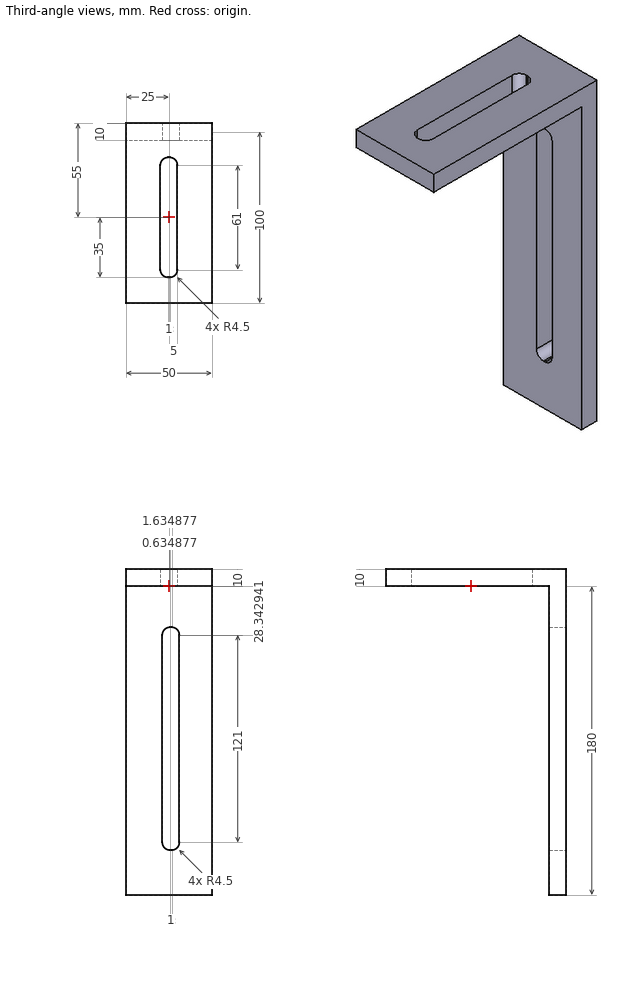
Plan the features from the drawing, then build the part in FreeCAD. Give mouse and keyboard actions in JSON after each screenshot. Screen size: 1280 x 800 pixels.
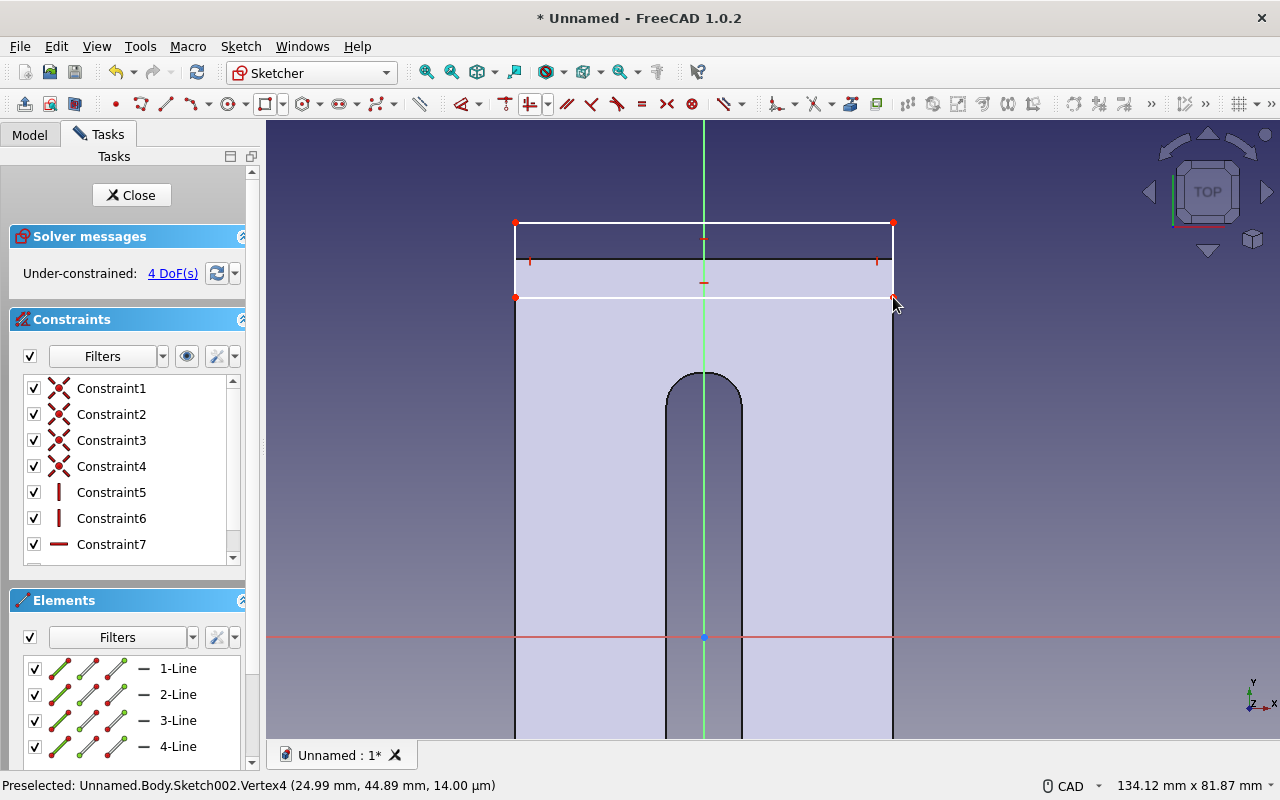
{"action": "left_click", "coordinate": [460, 104]}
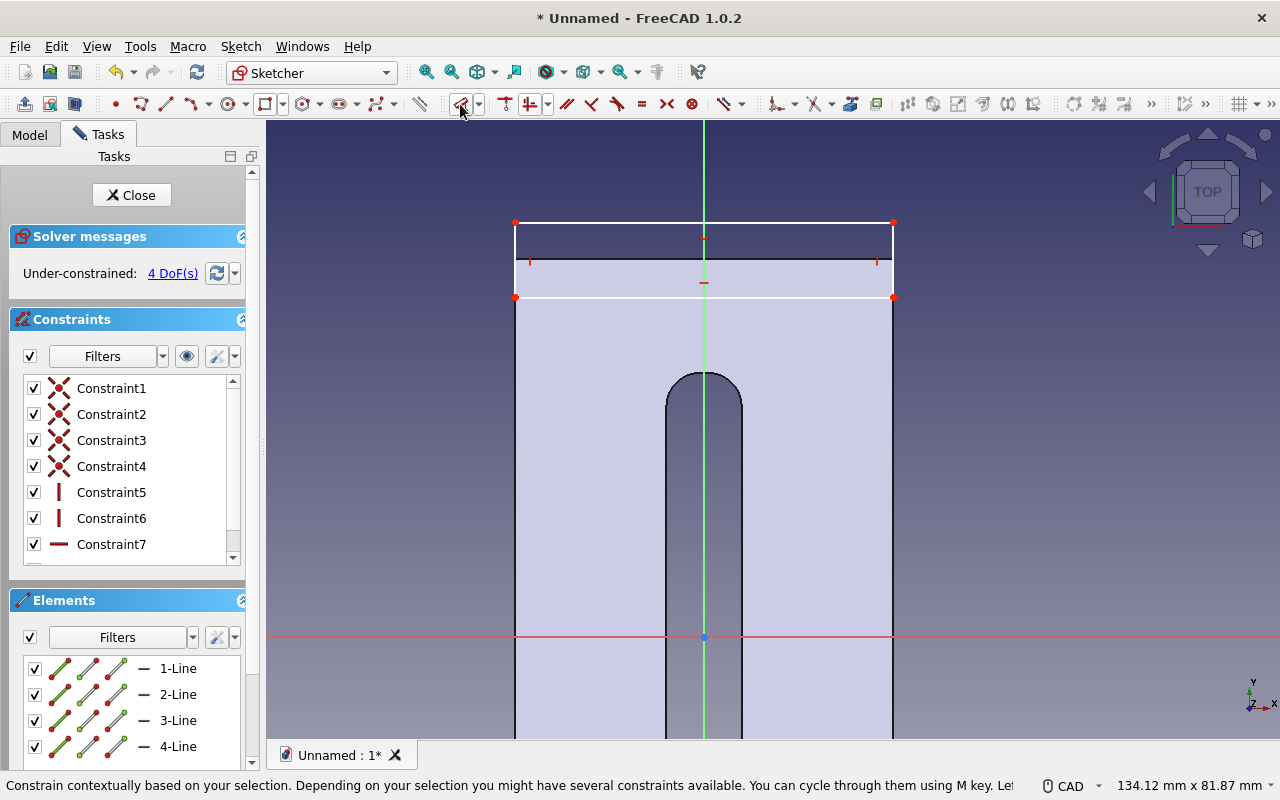
{"action": "left_click", "coordinate": [515, 245]}
{"action": "left_click", "coordinate": [481, 260]}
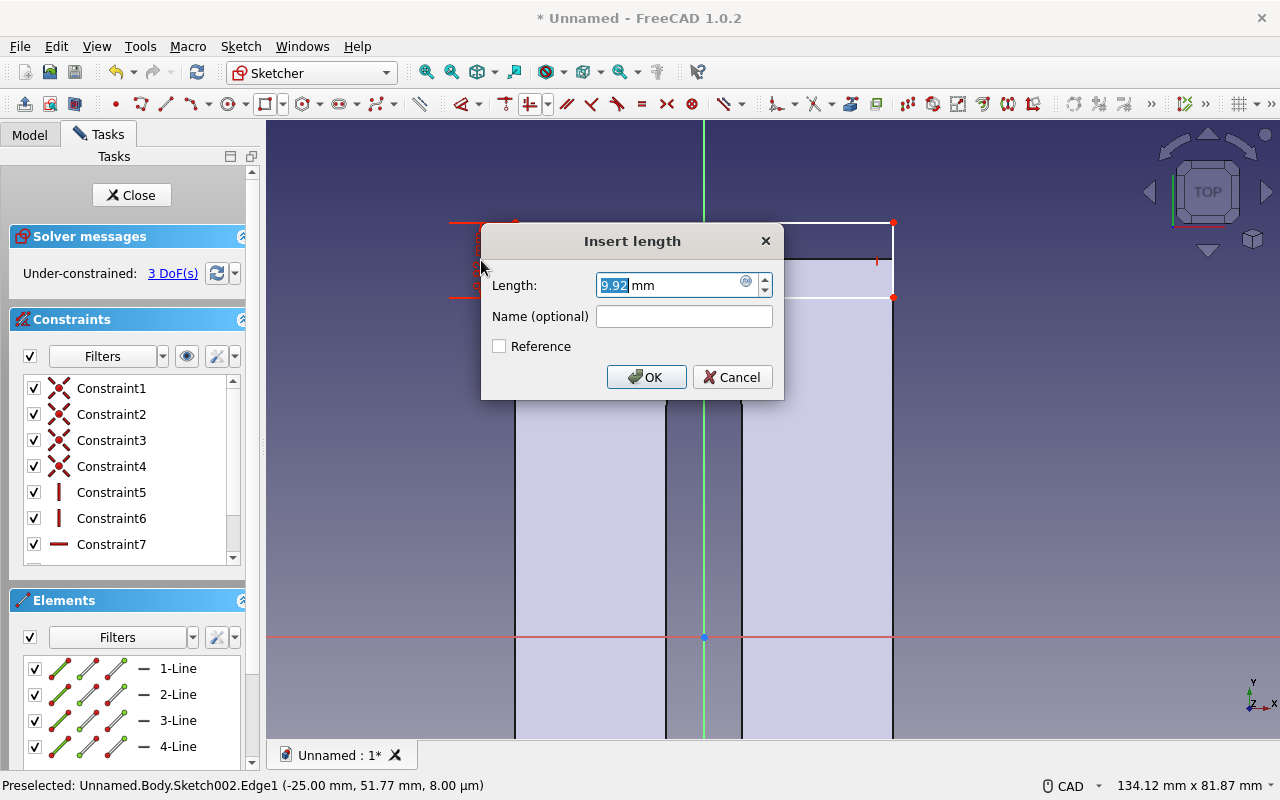
{"action": "type", "text": "10"}
{"action": "key", "text": "Return"}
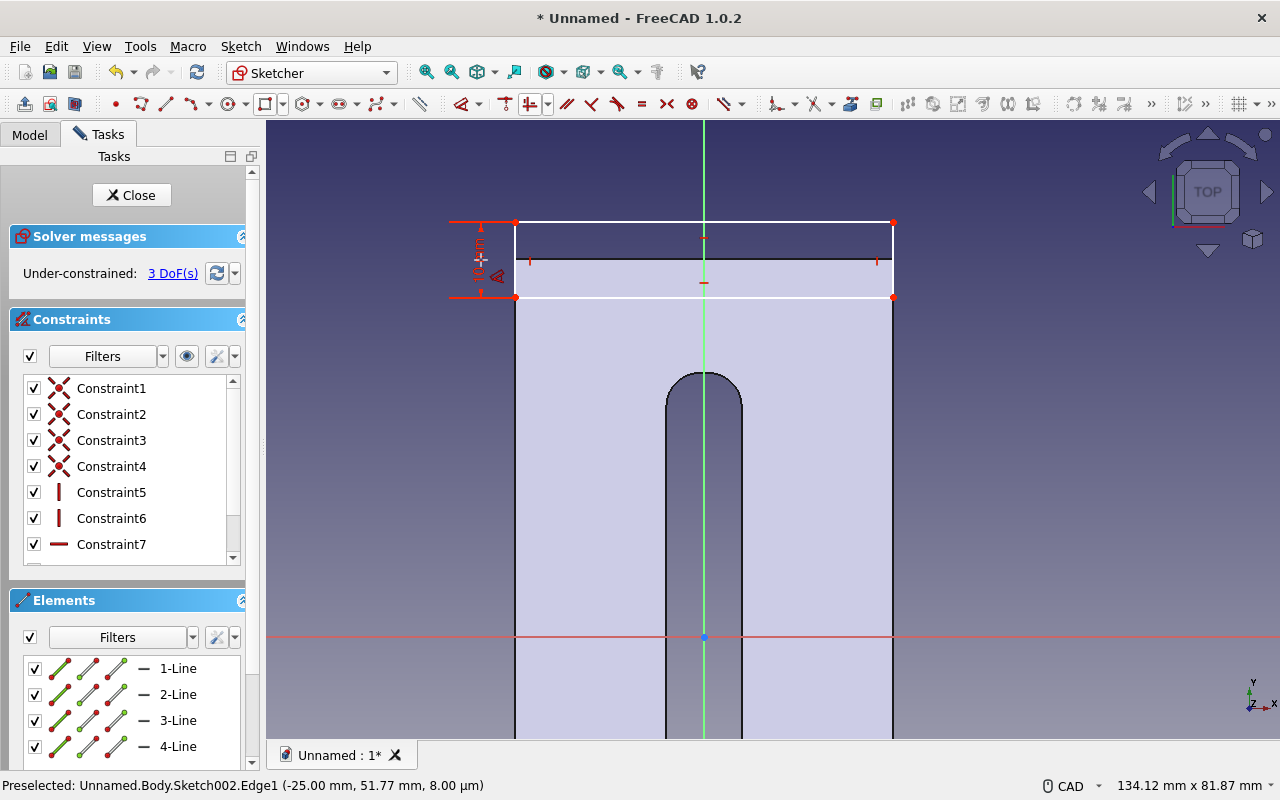
{"action": "left_click", "coordinate": [628, 298]}
{"action": "left_click", "coordinate": [617, 264]}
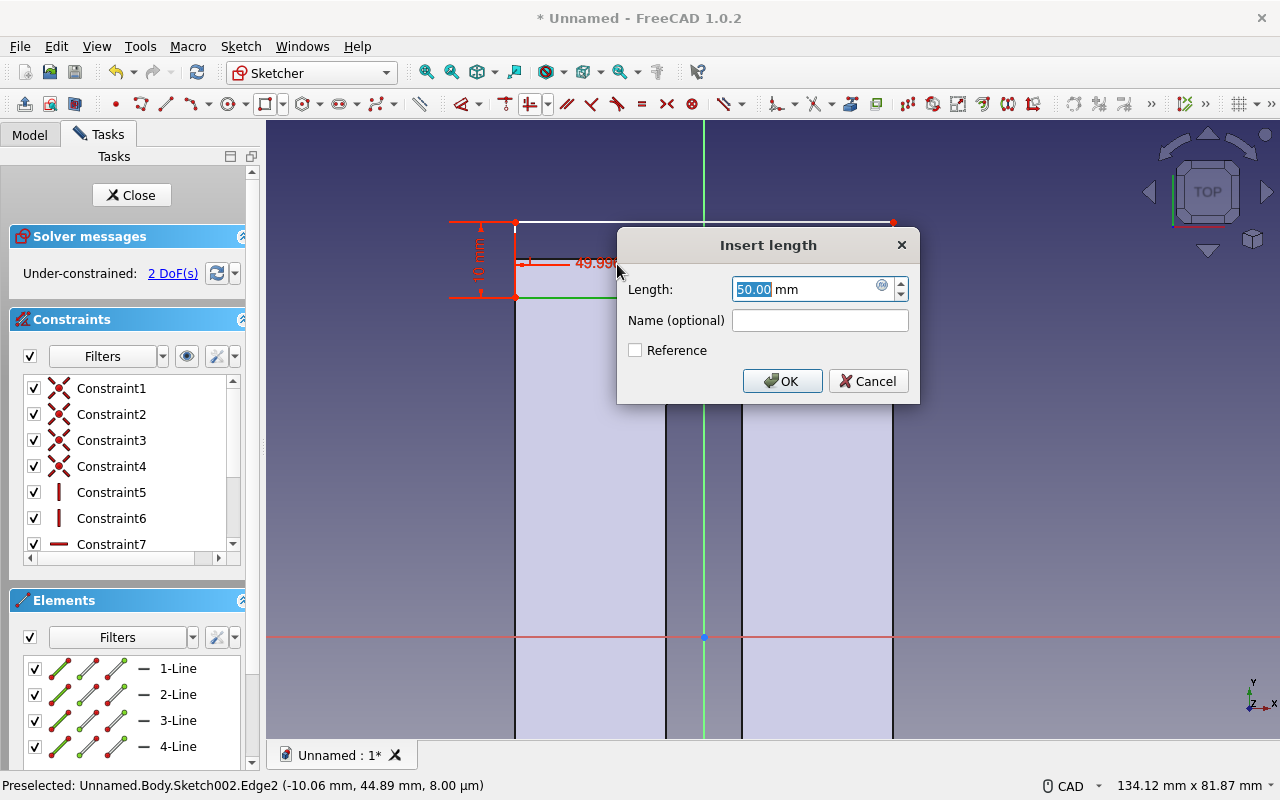
{"action": "type", "text": "50"}
{"action": "key", "text": "Return"}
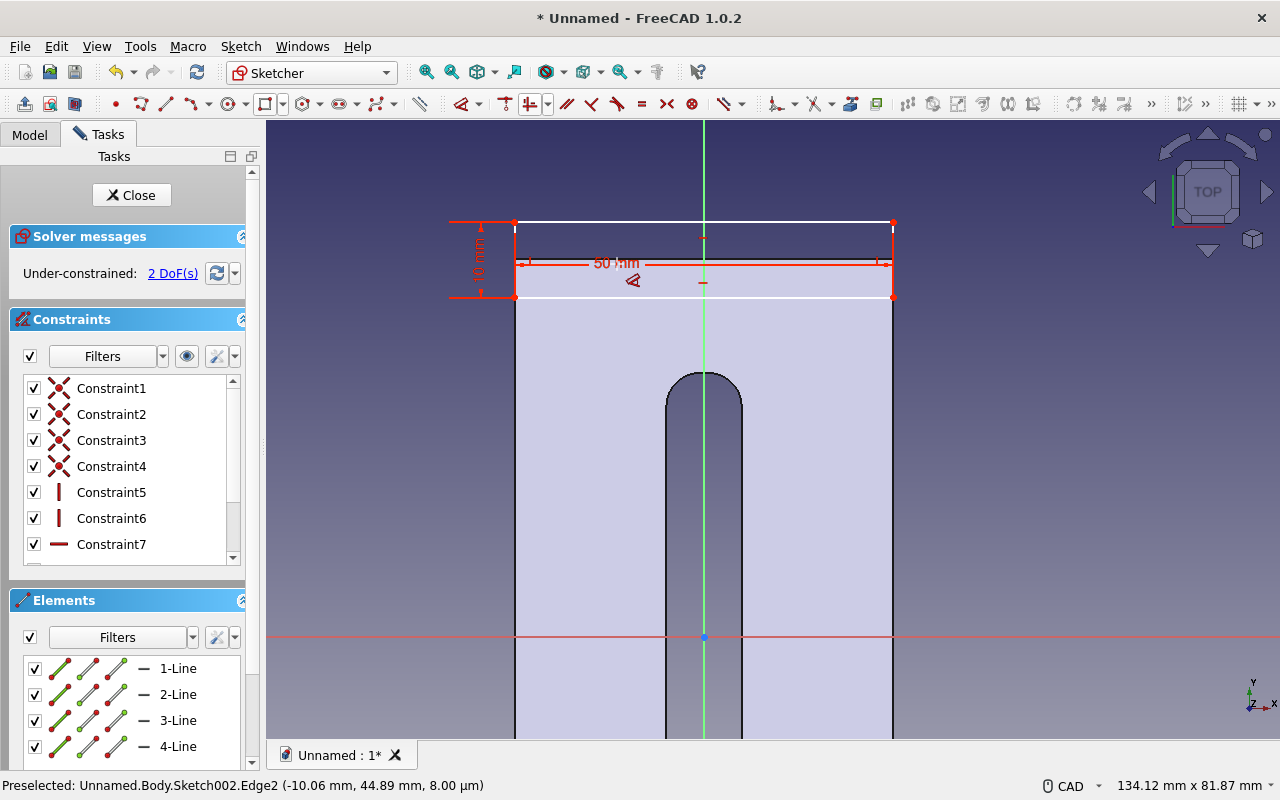
{"action": "left_click", "coordinate": [515, 222]}
{"action": "left_click", "coordinate": [610, 671]}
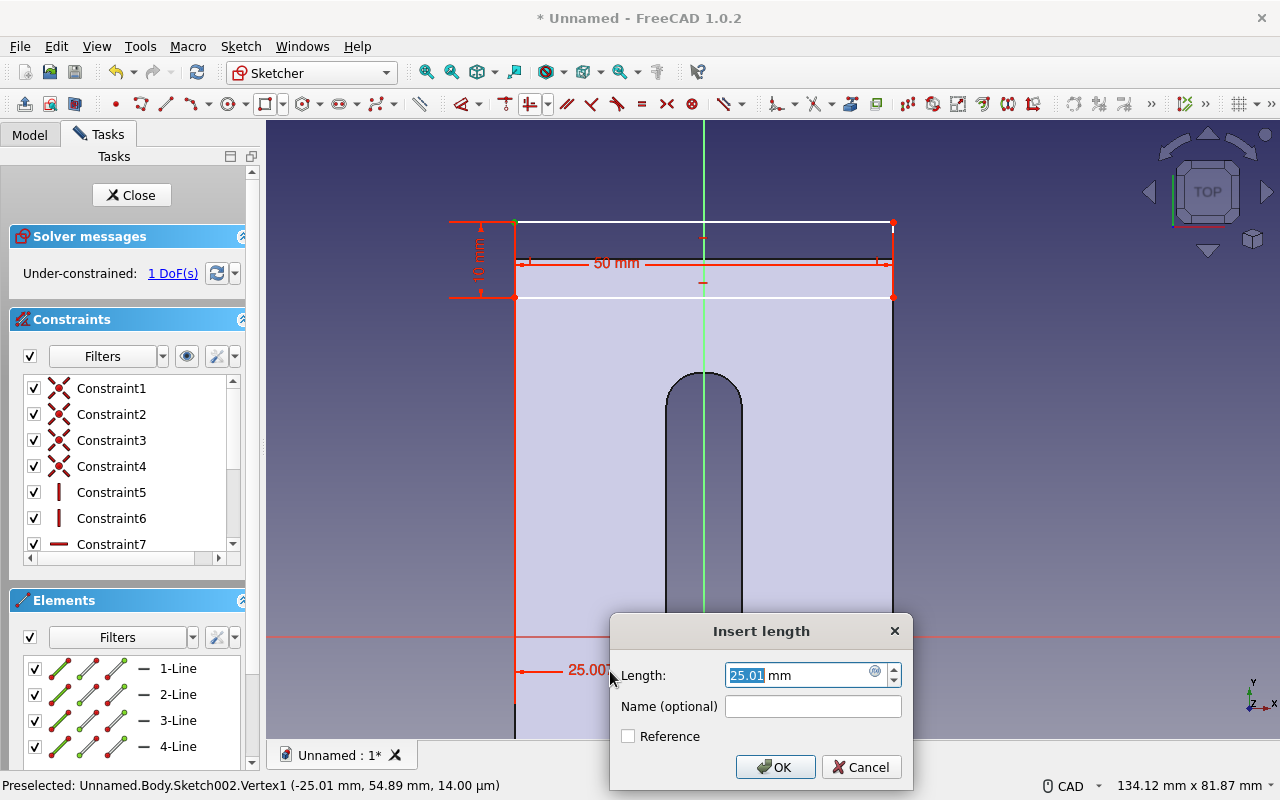
{"action": "type", "text": "25"}
{"action": "key", "text": "Return"}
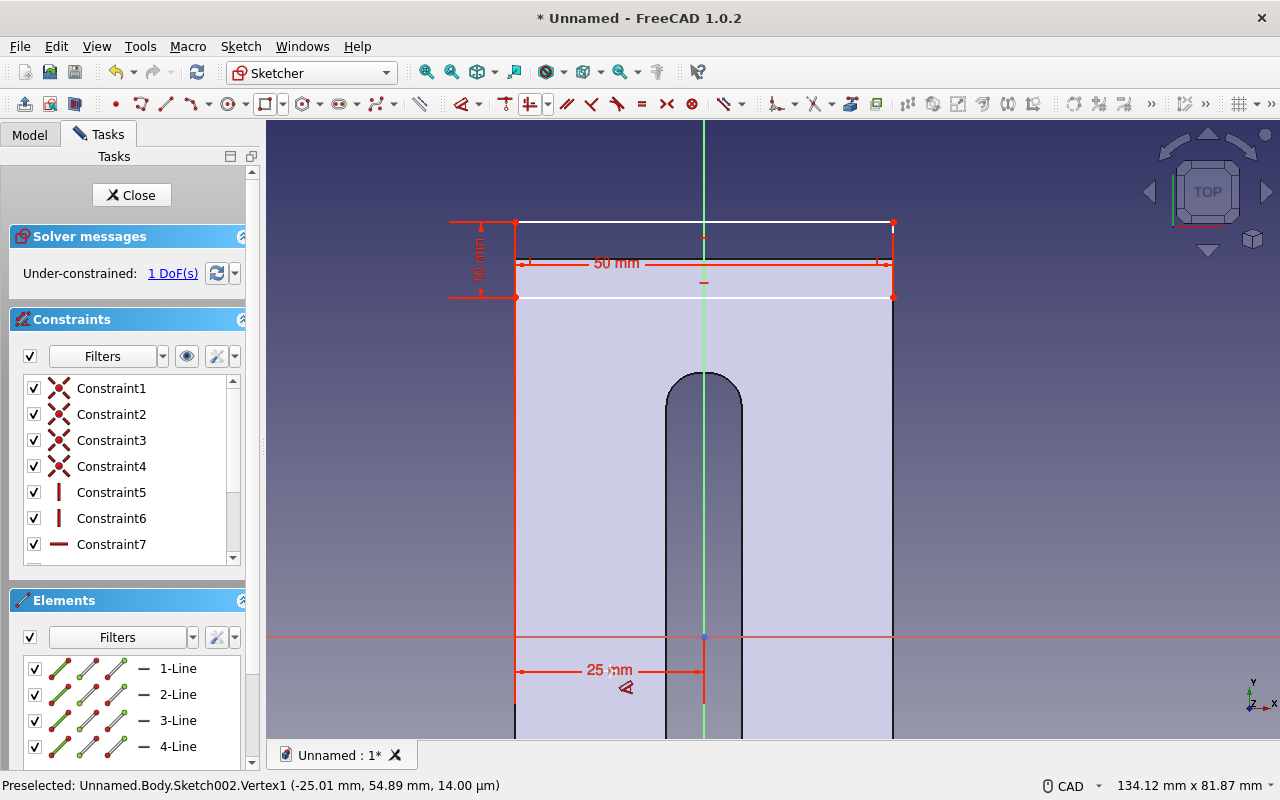
{"action": "left_click", "coordinate": [515, 222]}
{"action": "left_click", "coordinate": [481, 430]}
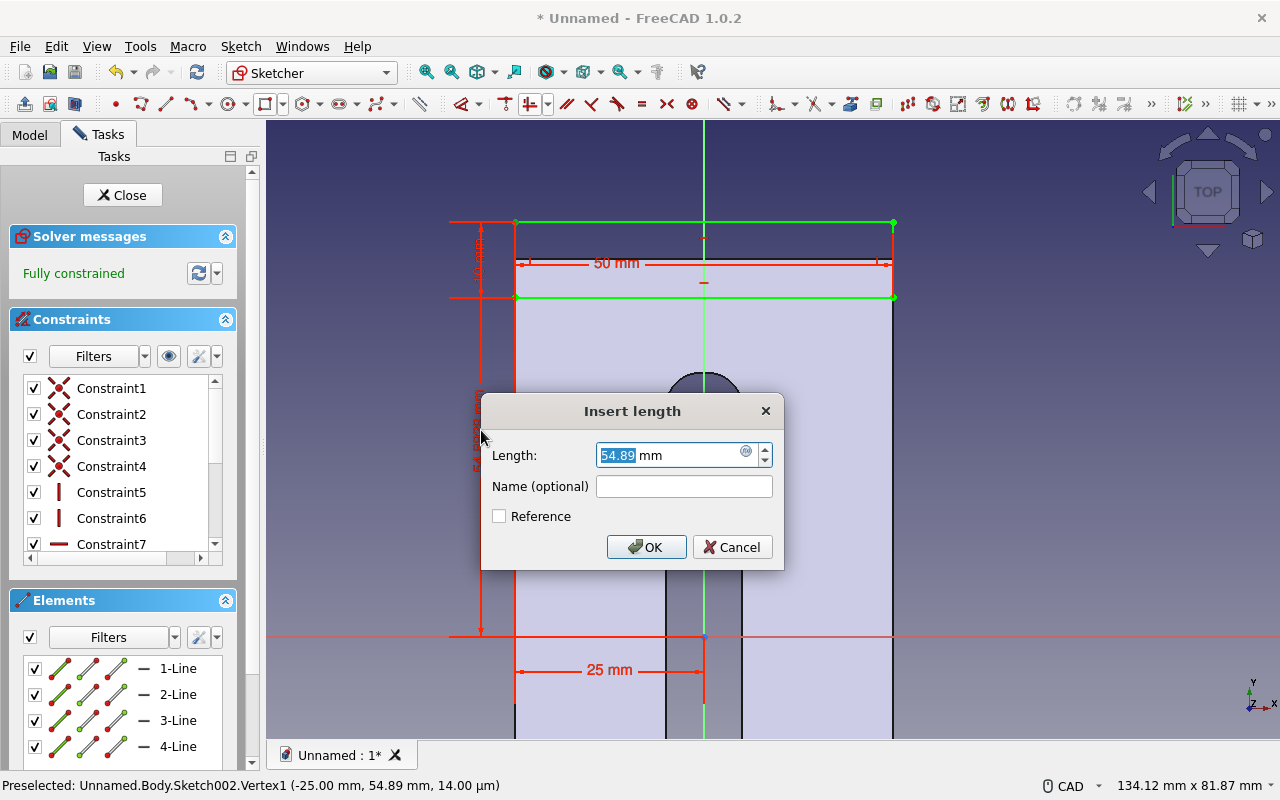
{"action": "type", "text": "55"}
{"action": "key", "text": "Return"}
{"action": "key", "text": "Escape"}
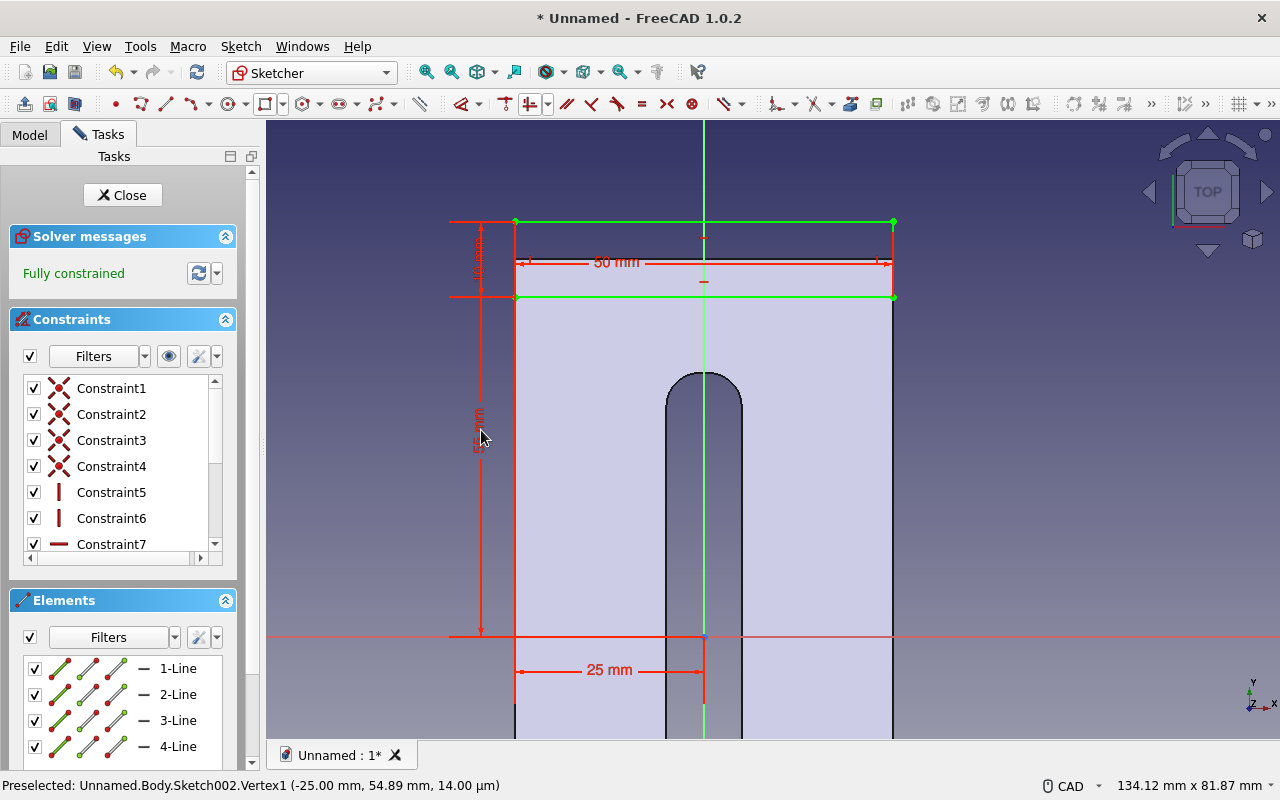
{"action": "left_click", "coordinate": [123, 195]}